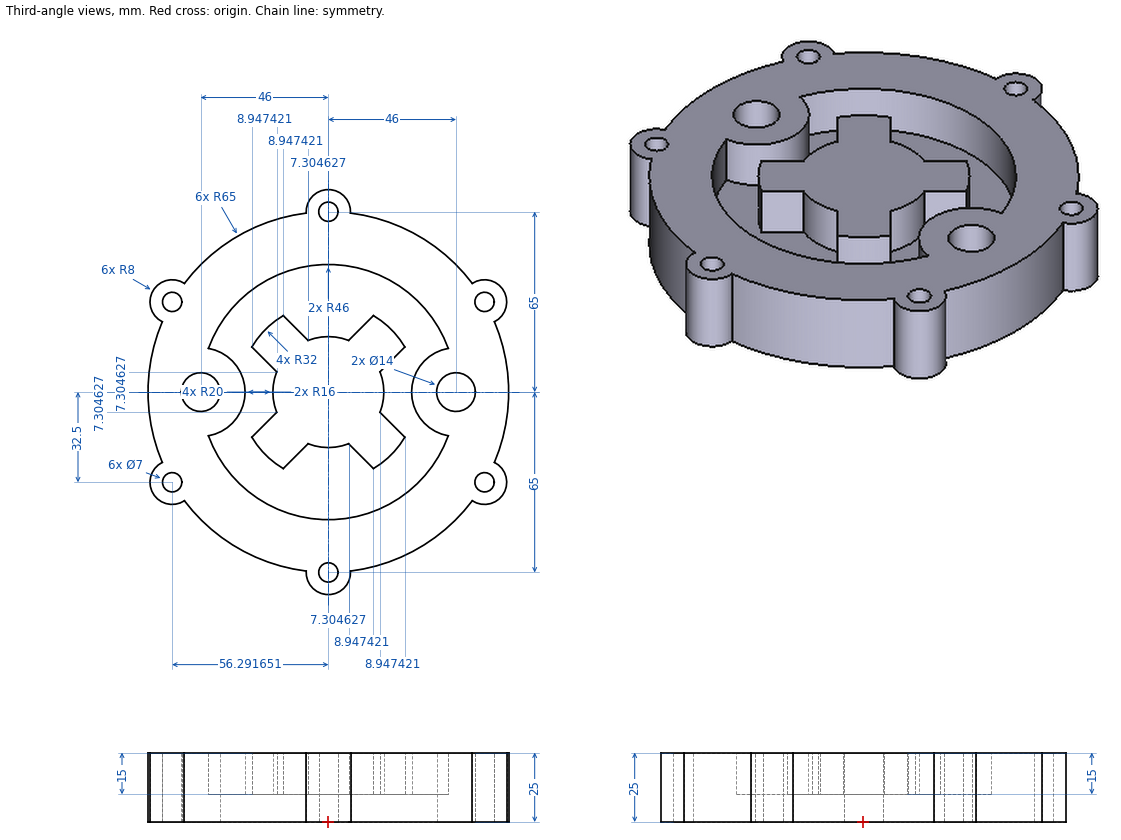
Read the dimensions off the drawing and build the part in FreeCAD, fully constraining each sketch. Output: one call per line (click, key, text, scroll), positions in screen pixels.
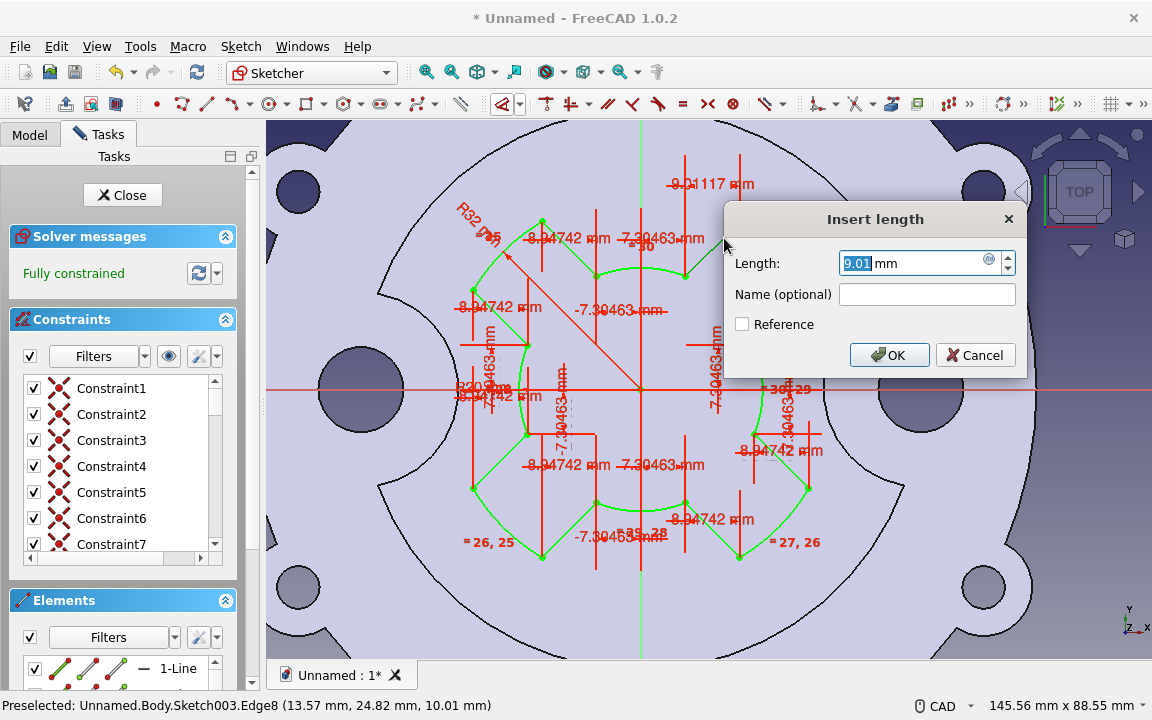
text(8.947421)
key(Return)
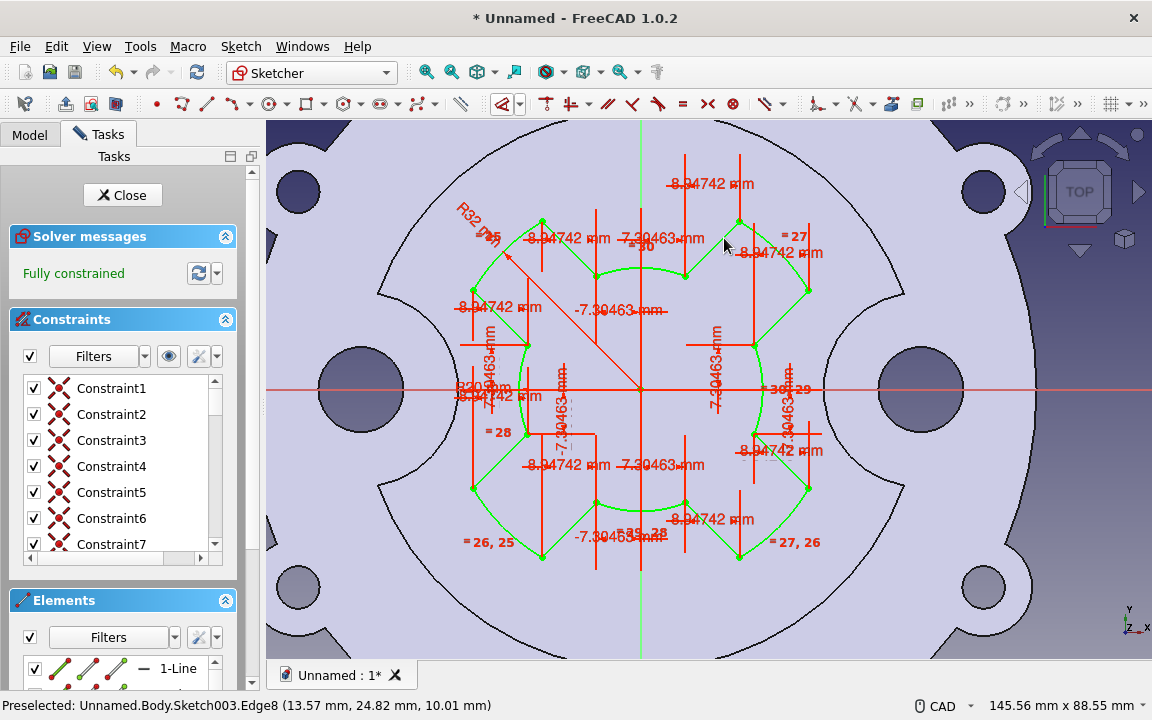
click(123, 195)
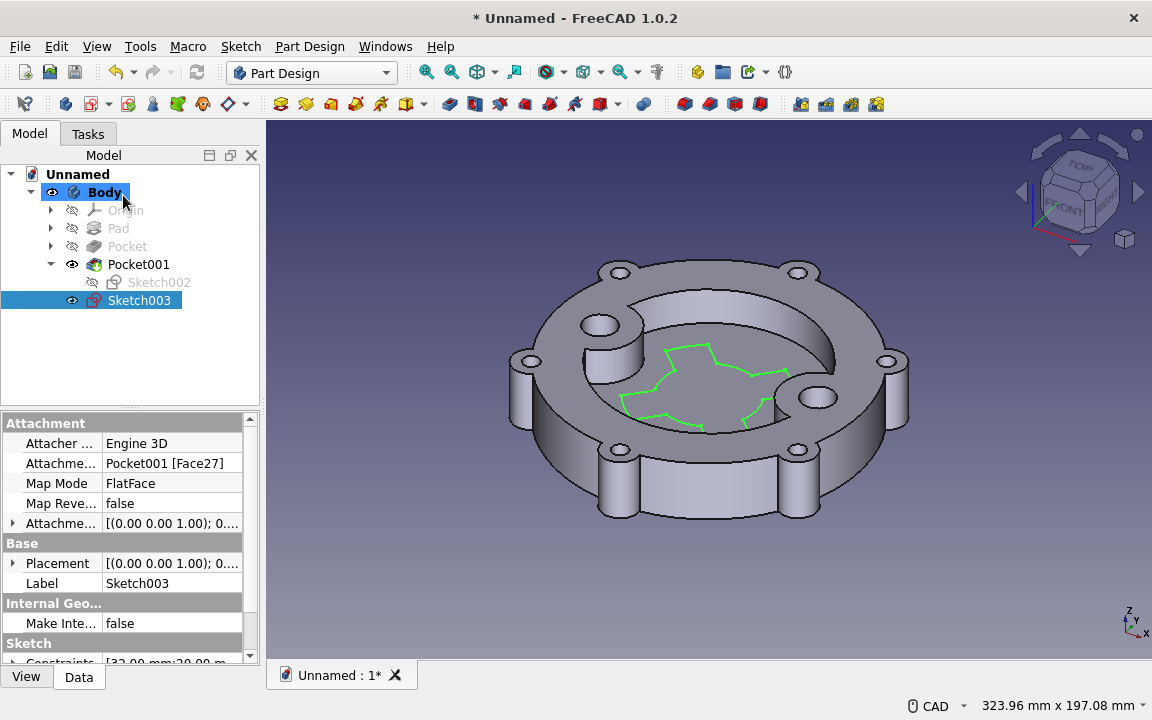
click(281, 104)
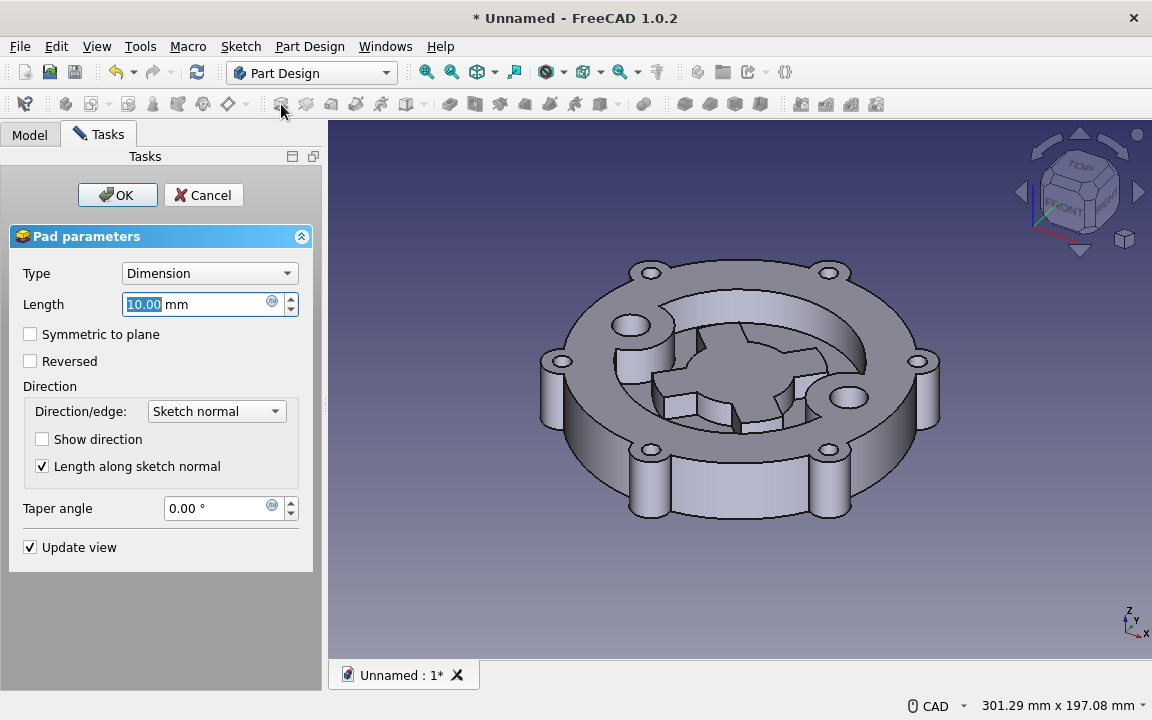
text(15)
key(Tab)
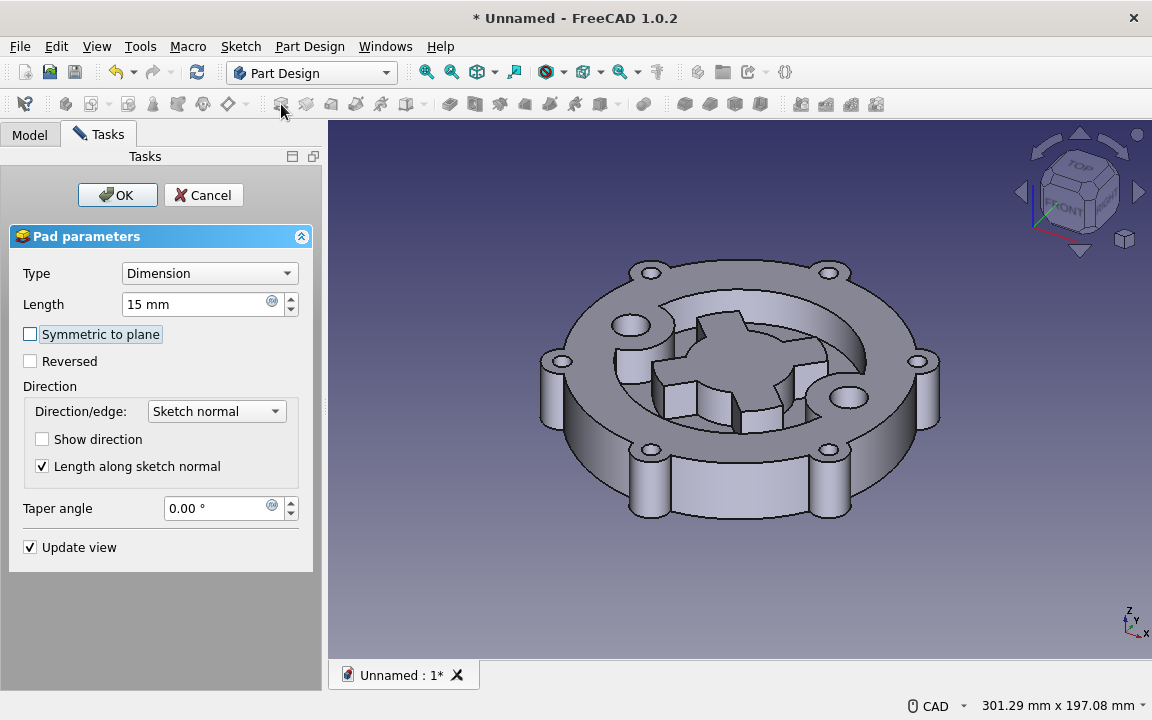
click(118, 195)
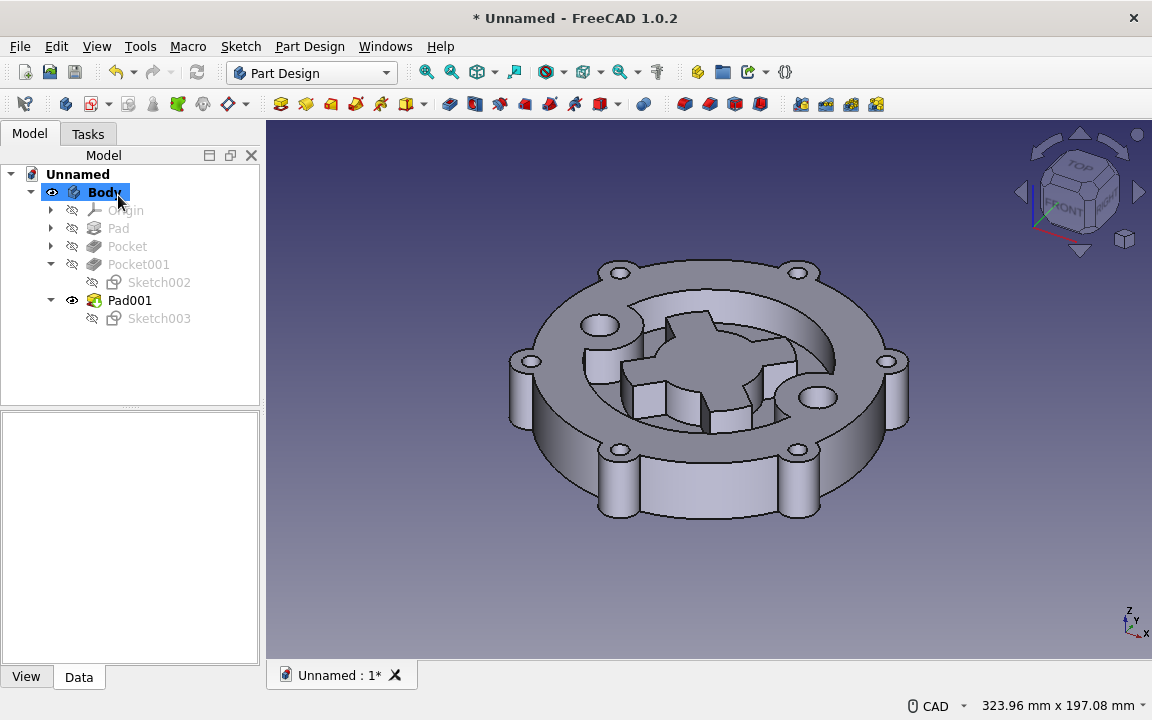
key(0)